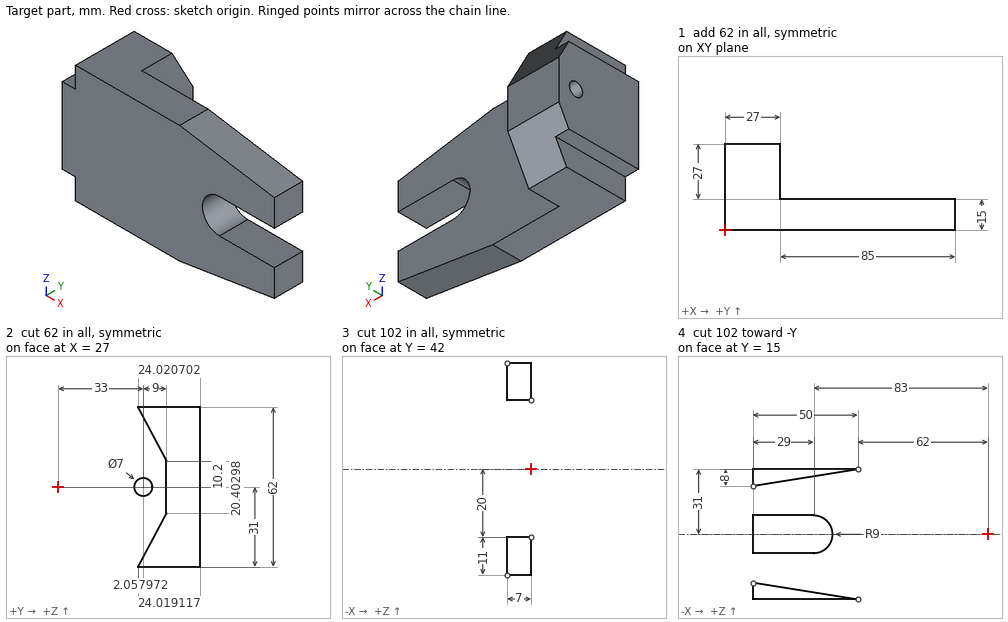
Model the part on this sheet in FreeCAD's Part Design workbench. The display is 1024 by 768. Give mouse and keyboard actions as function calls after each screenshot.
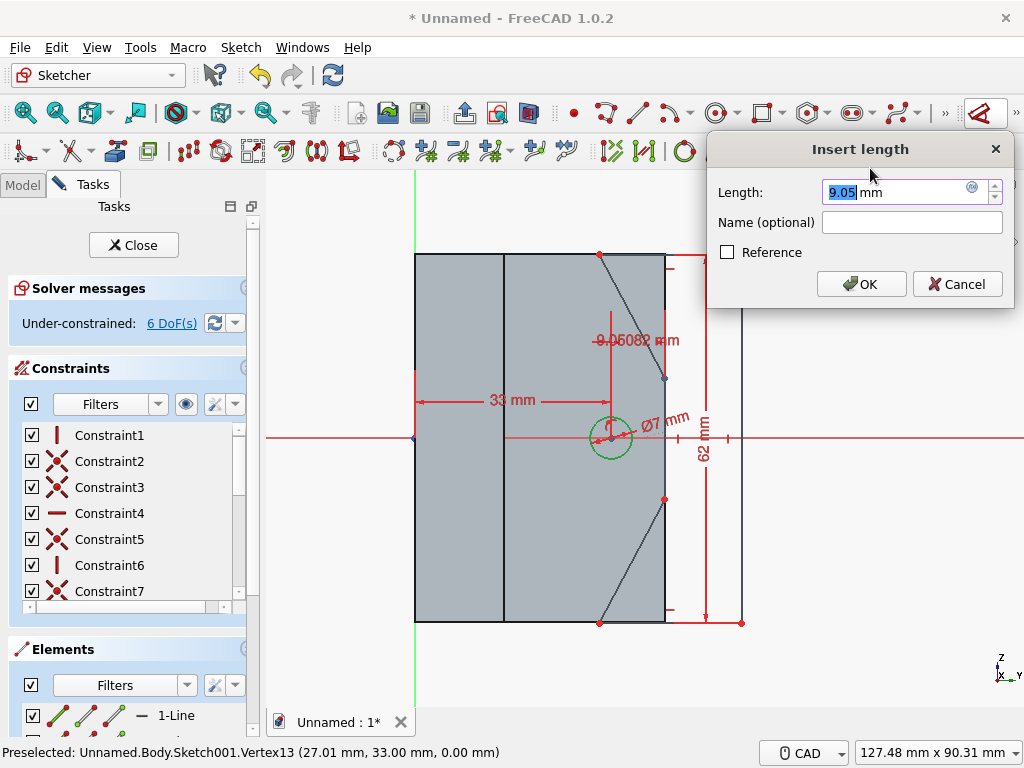
text(9)
key(Return)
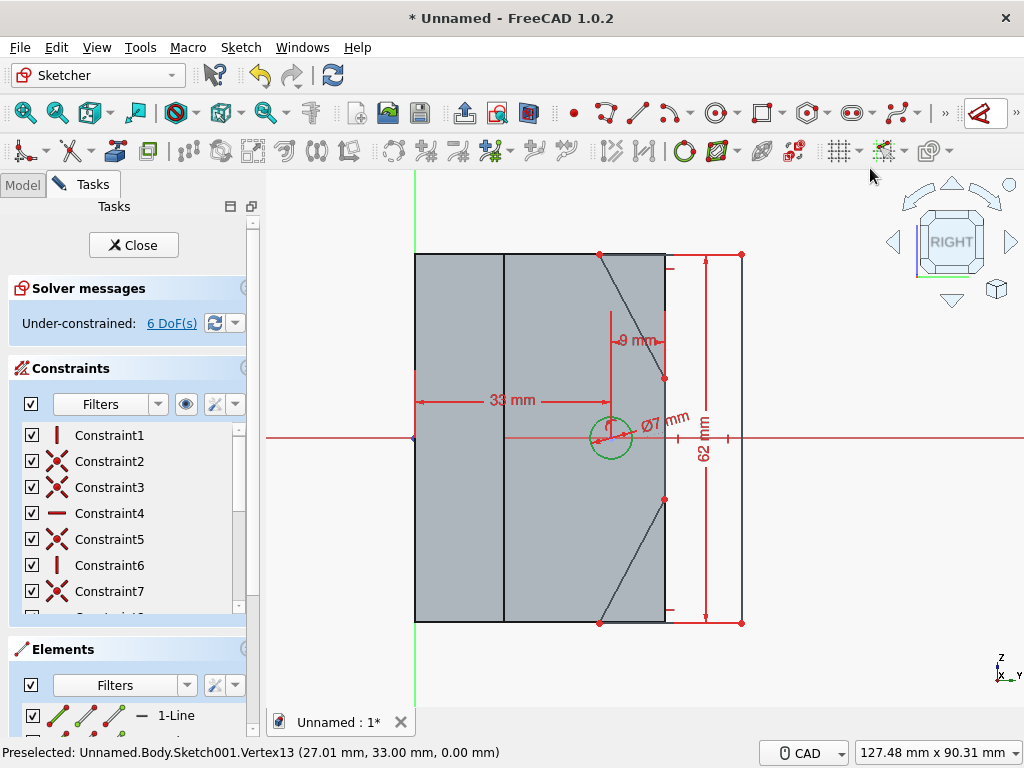
click(599, 623)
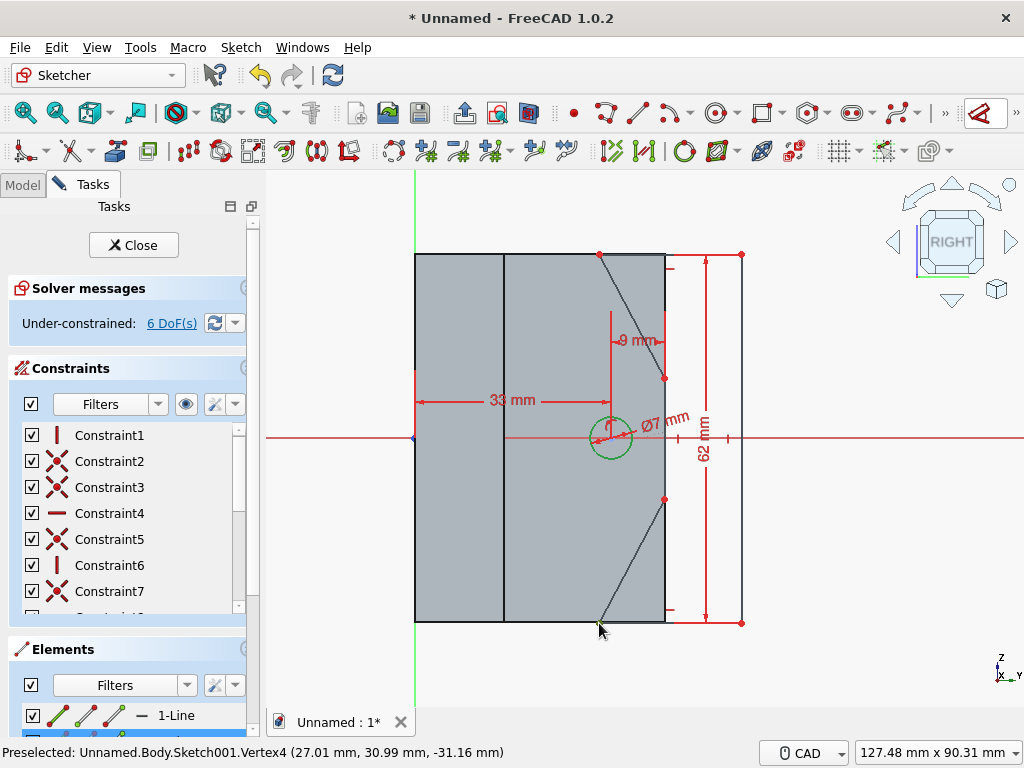
key(i)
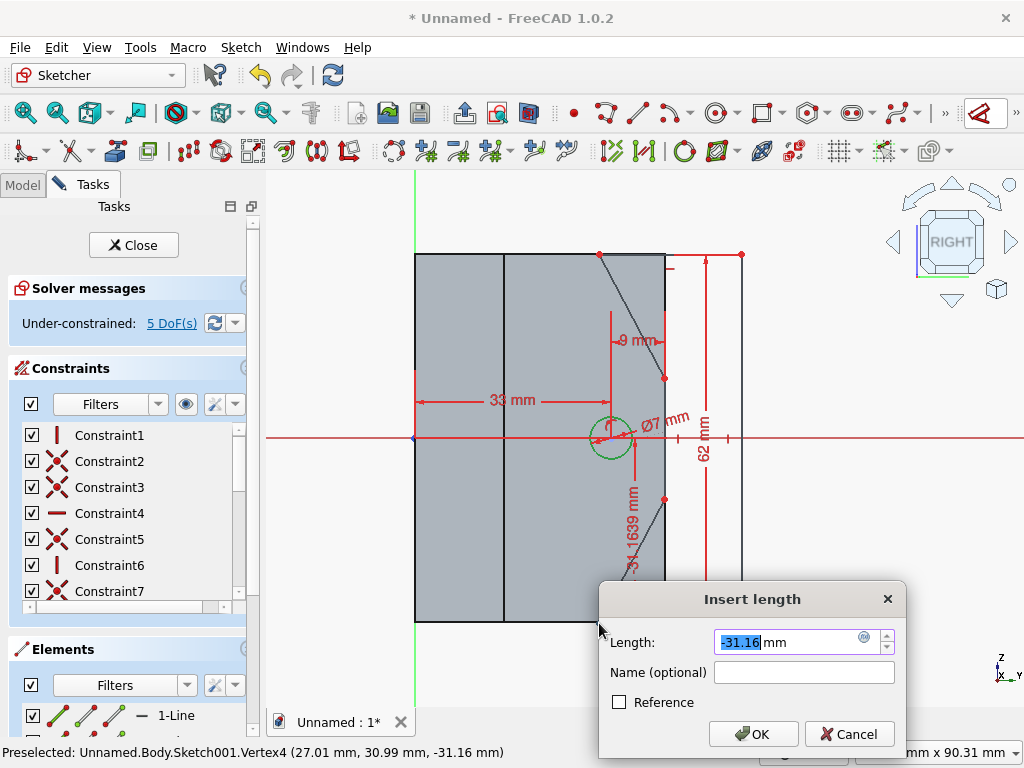
text(-31)
key(Return)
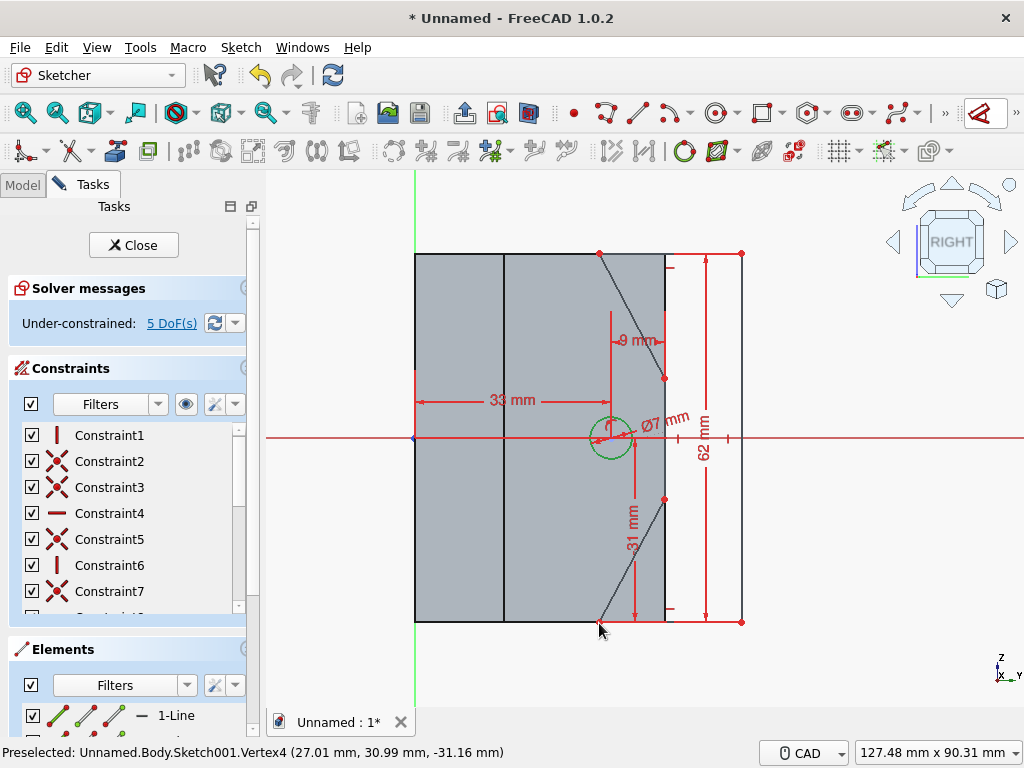
click(665, 378)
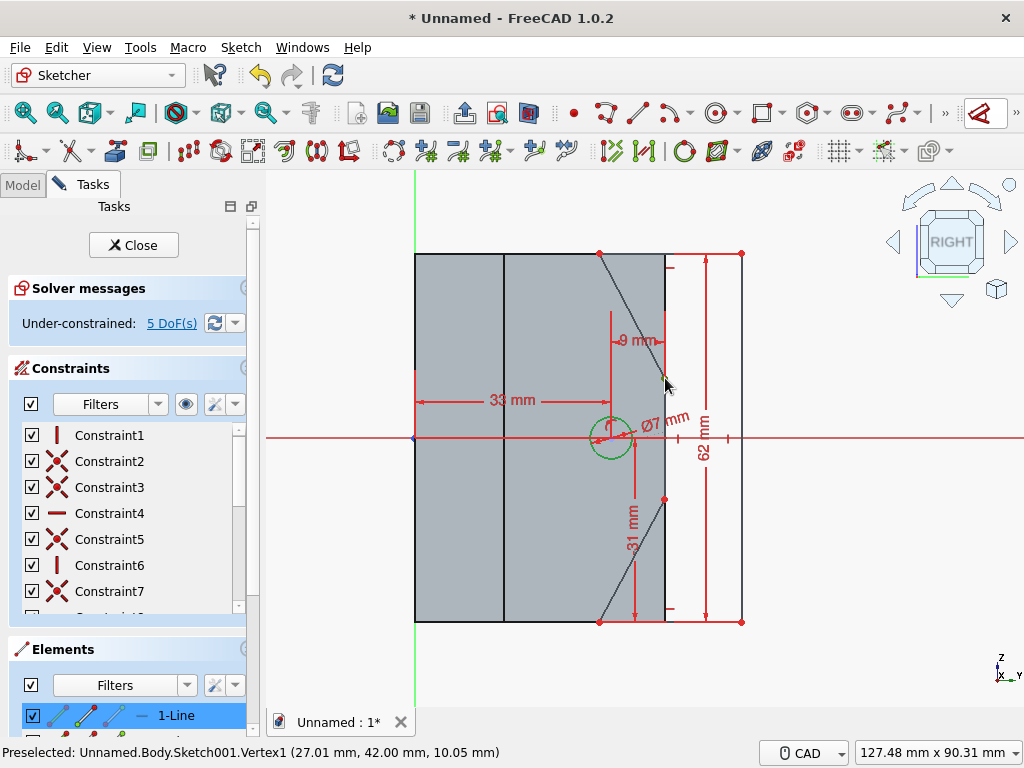
key(i)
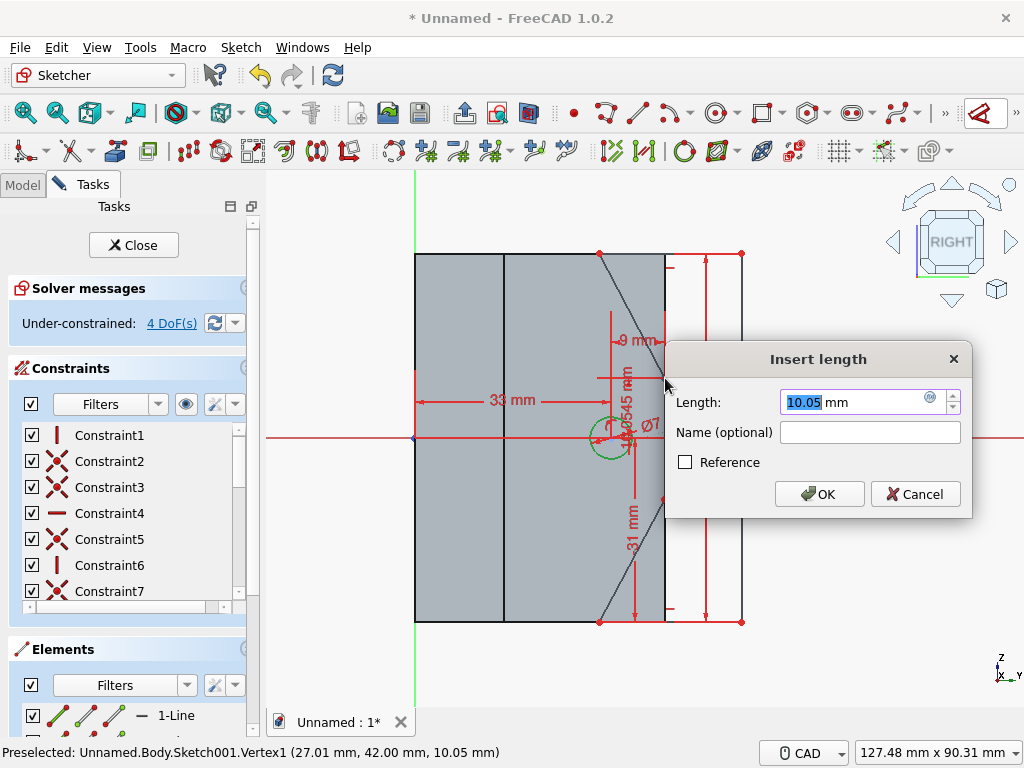
text(10.2)
key(Return)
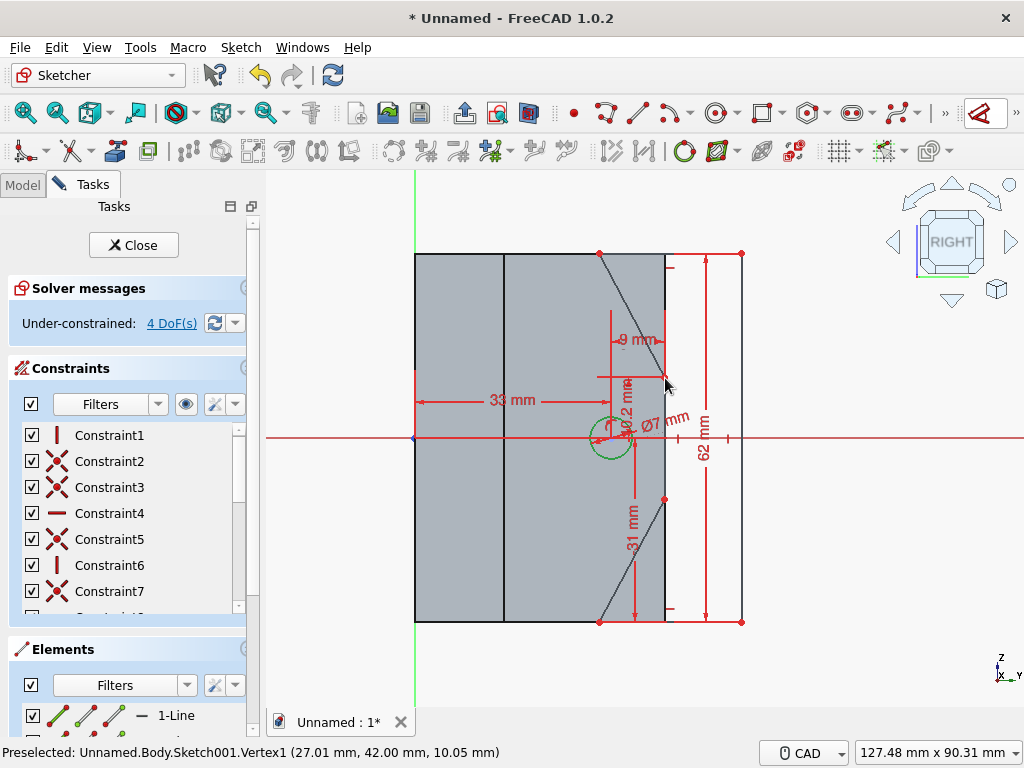
click(665, 414)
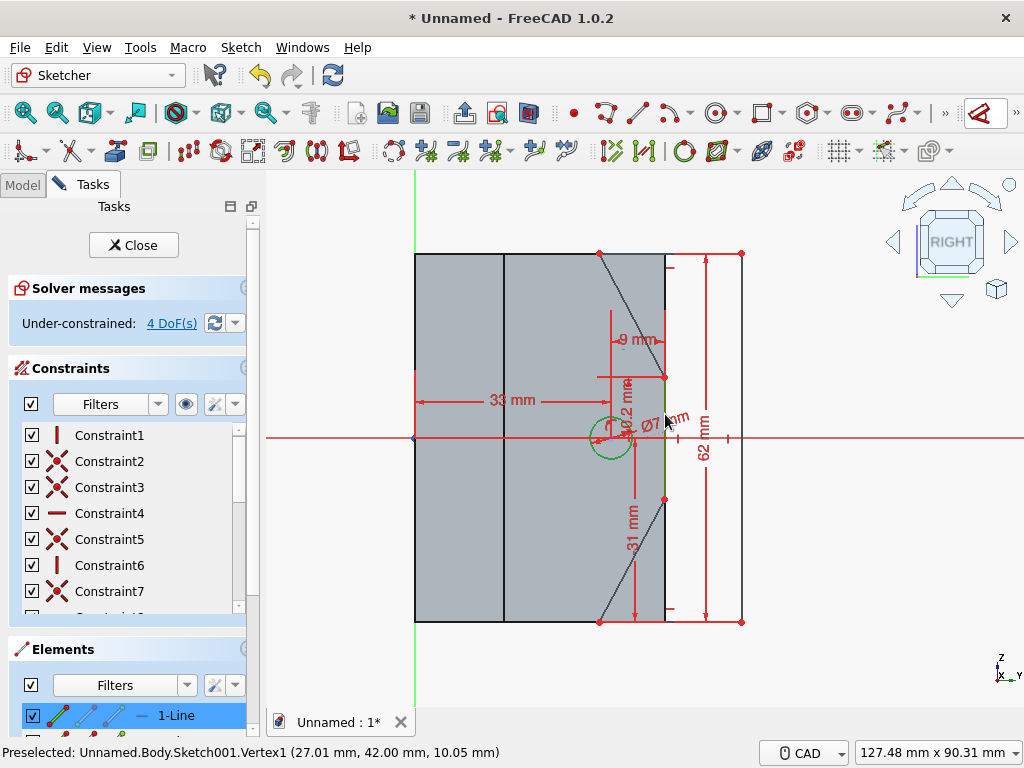
key(i)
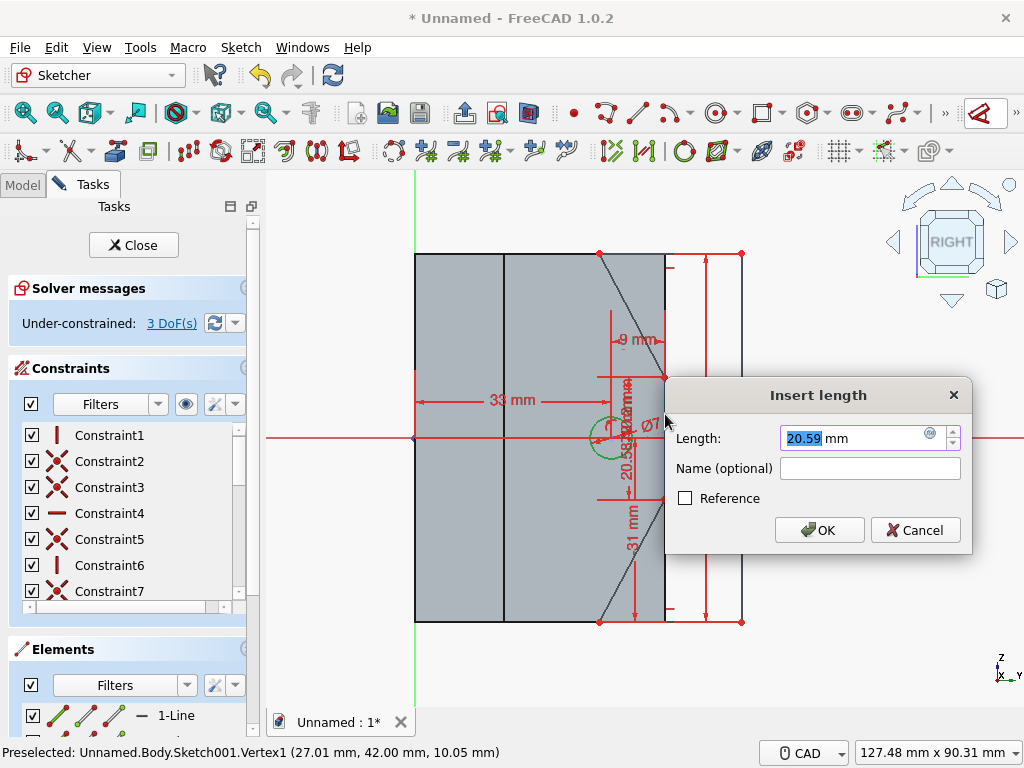
text(20.40298)
key(Return)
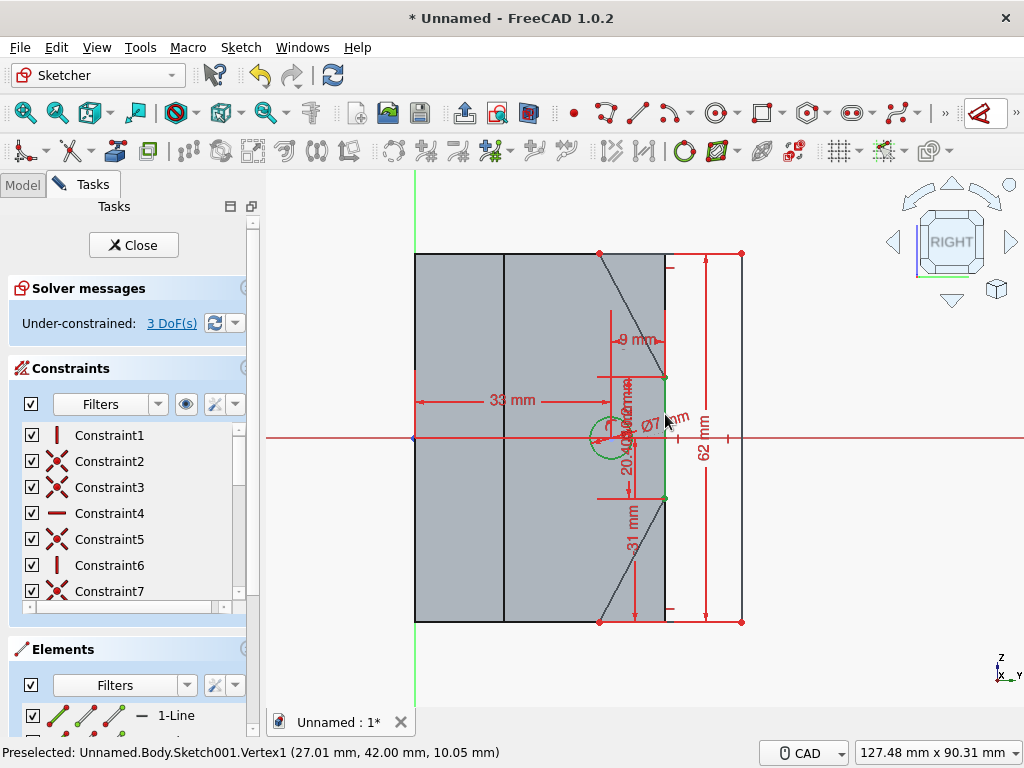
click(642, 622)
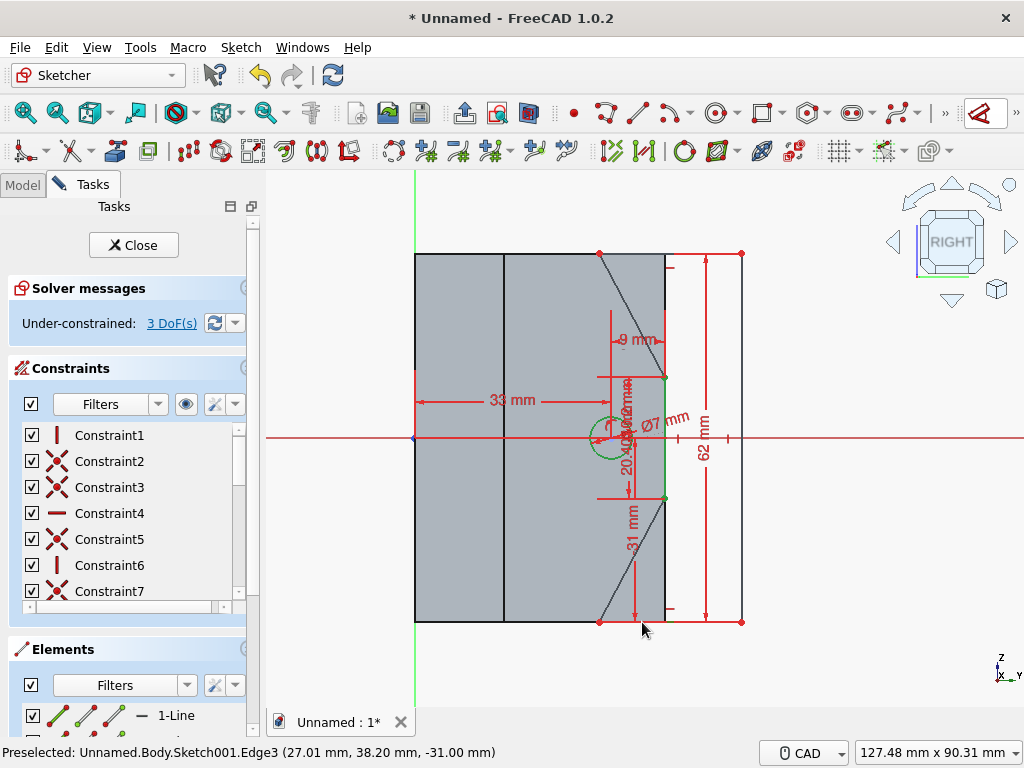
key(l)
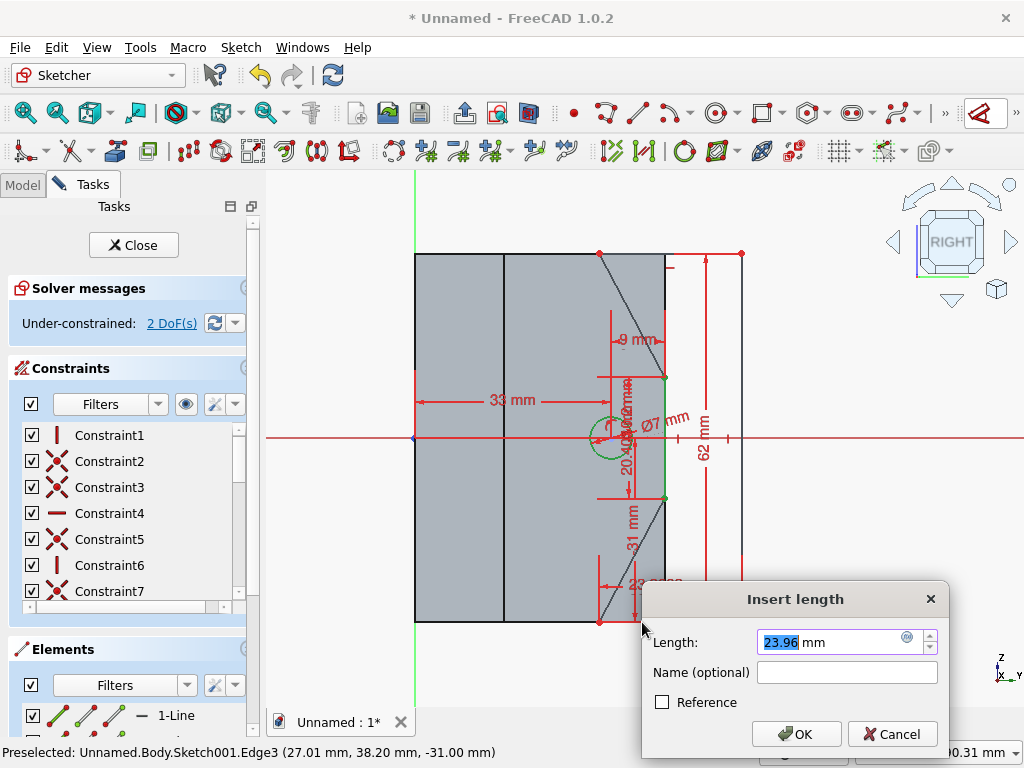
text(24.019117)
key(Return)